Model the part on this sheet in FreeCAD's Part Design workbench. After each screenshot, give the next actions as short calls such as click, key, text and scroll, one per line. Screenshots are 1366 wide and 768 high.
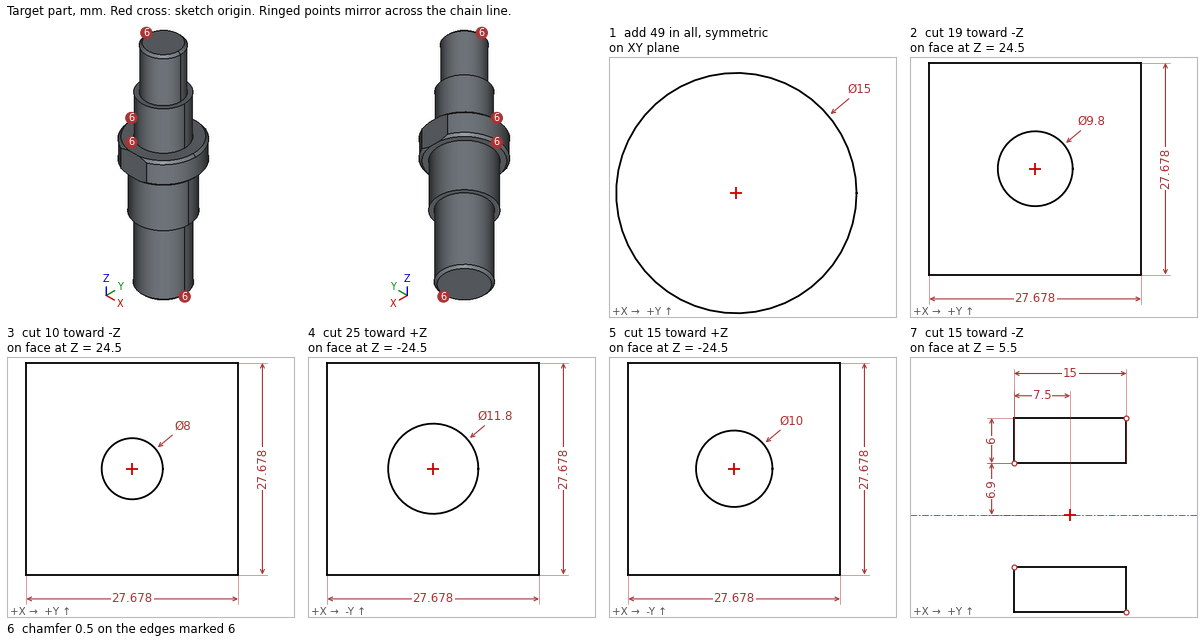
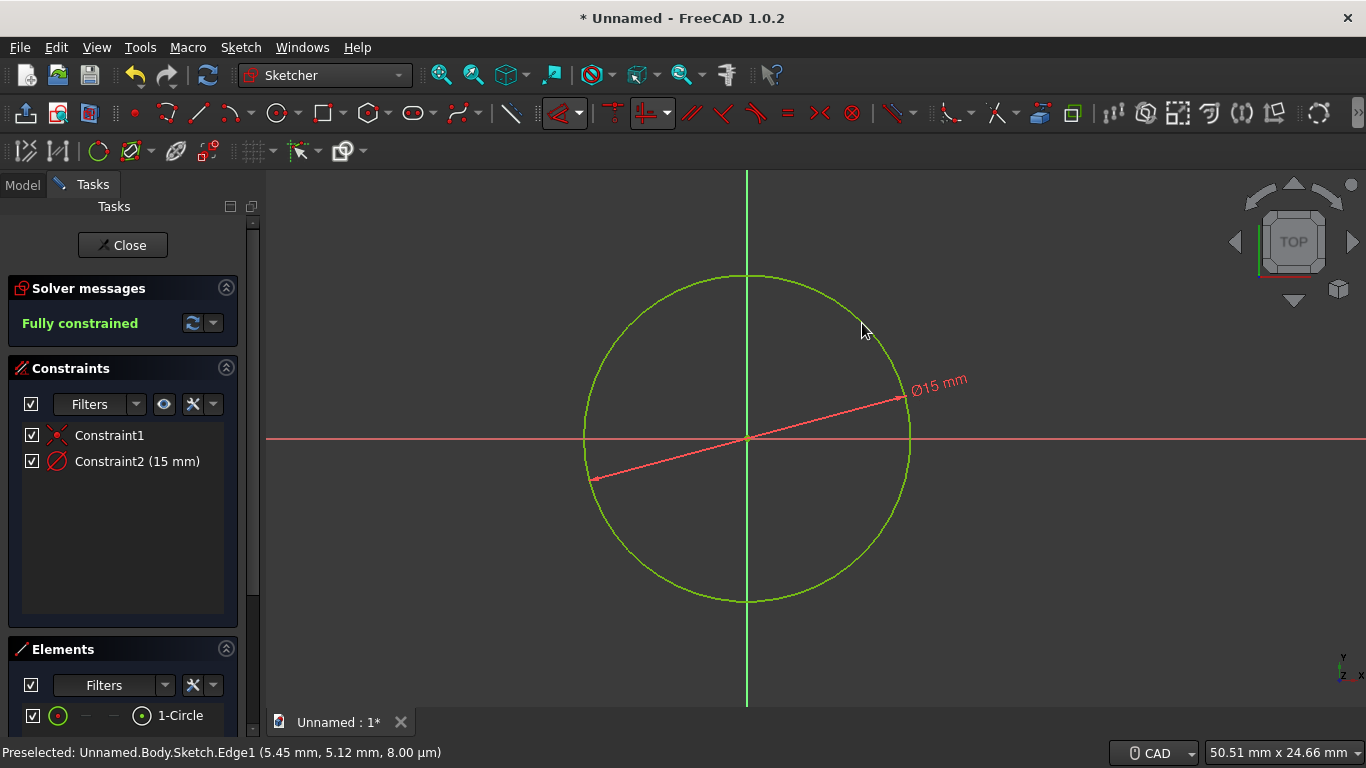
click(123, 245)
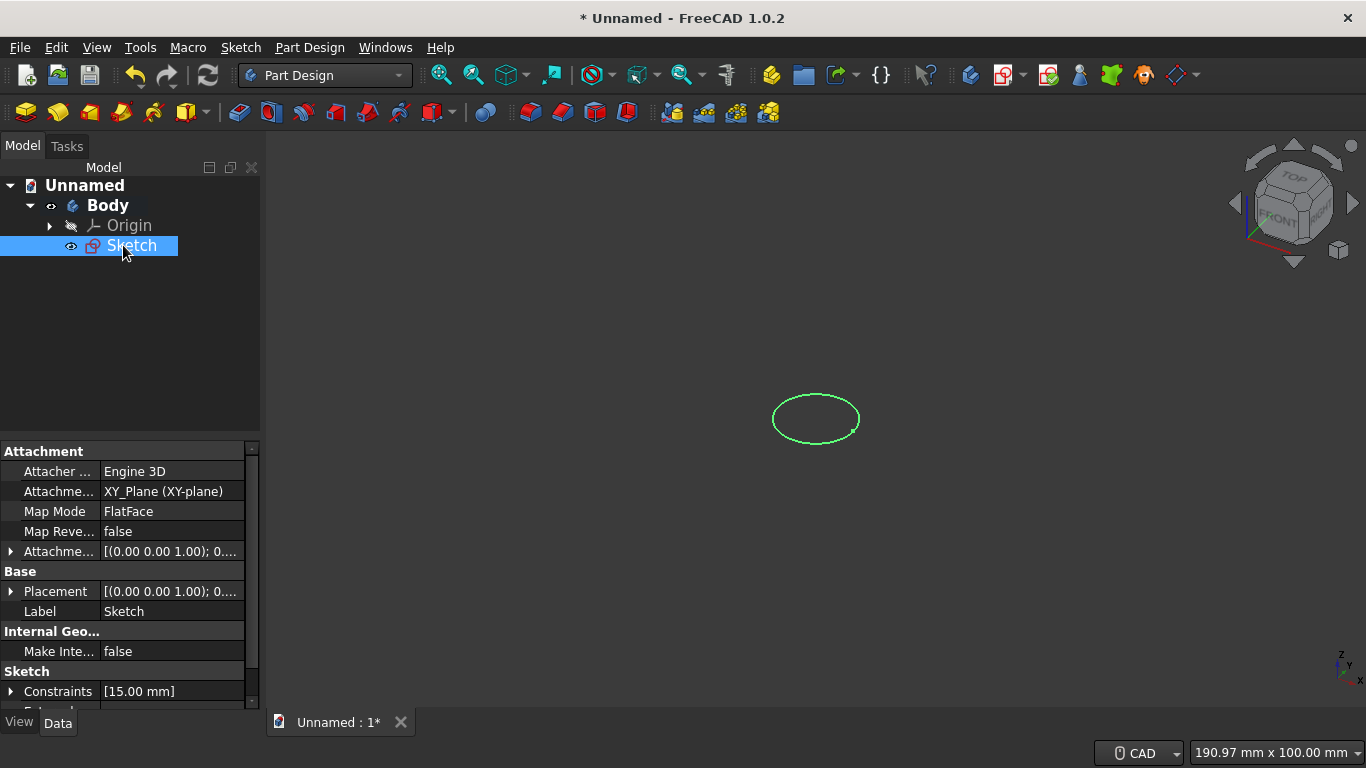
click(26, 112)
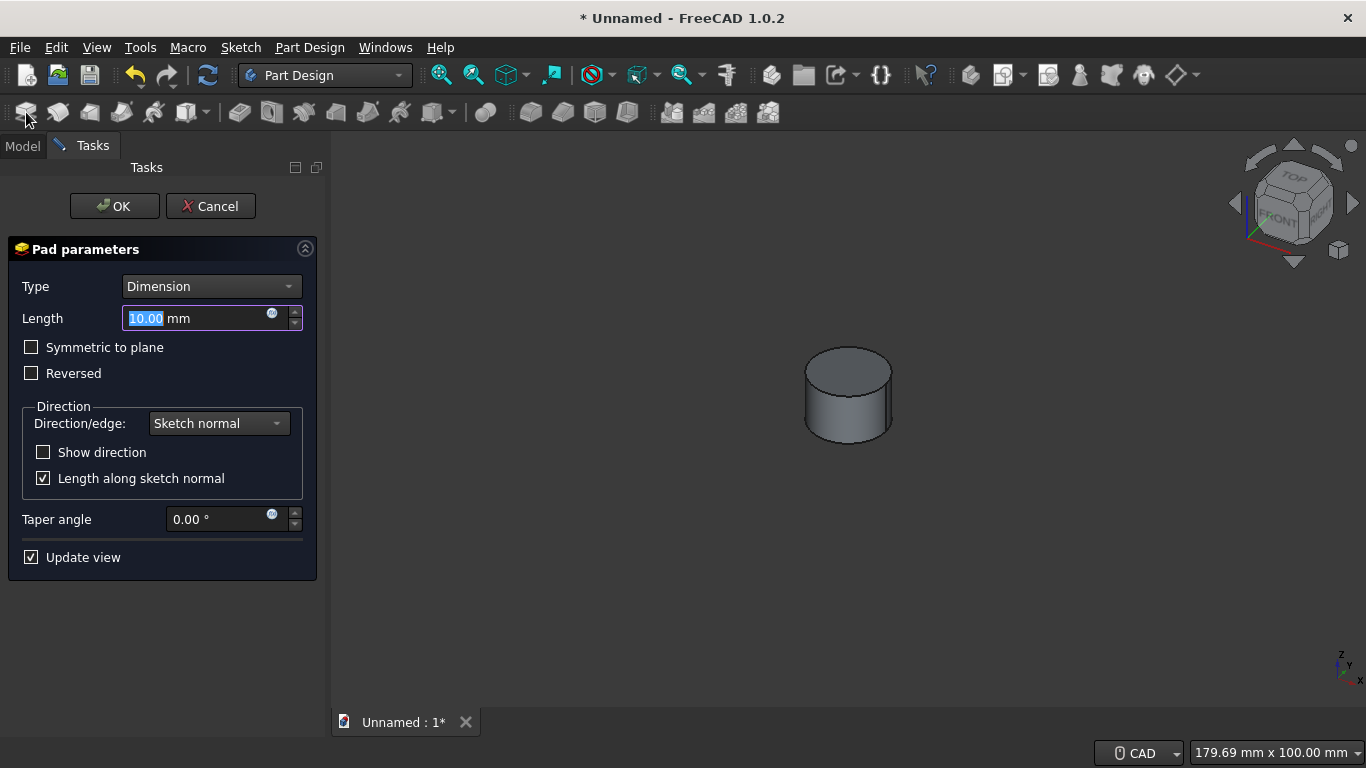
text(49)
key(Tab)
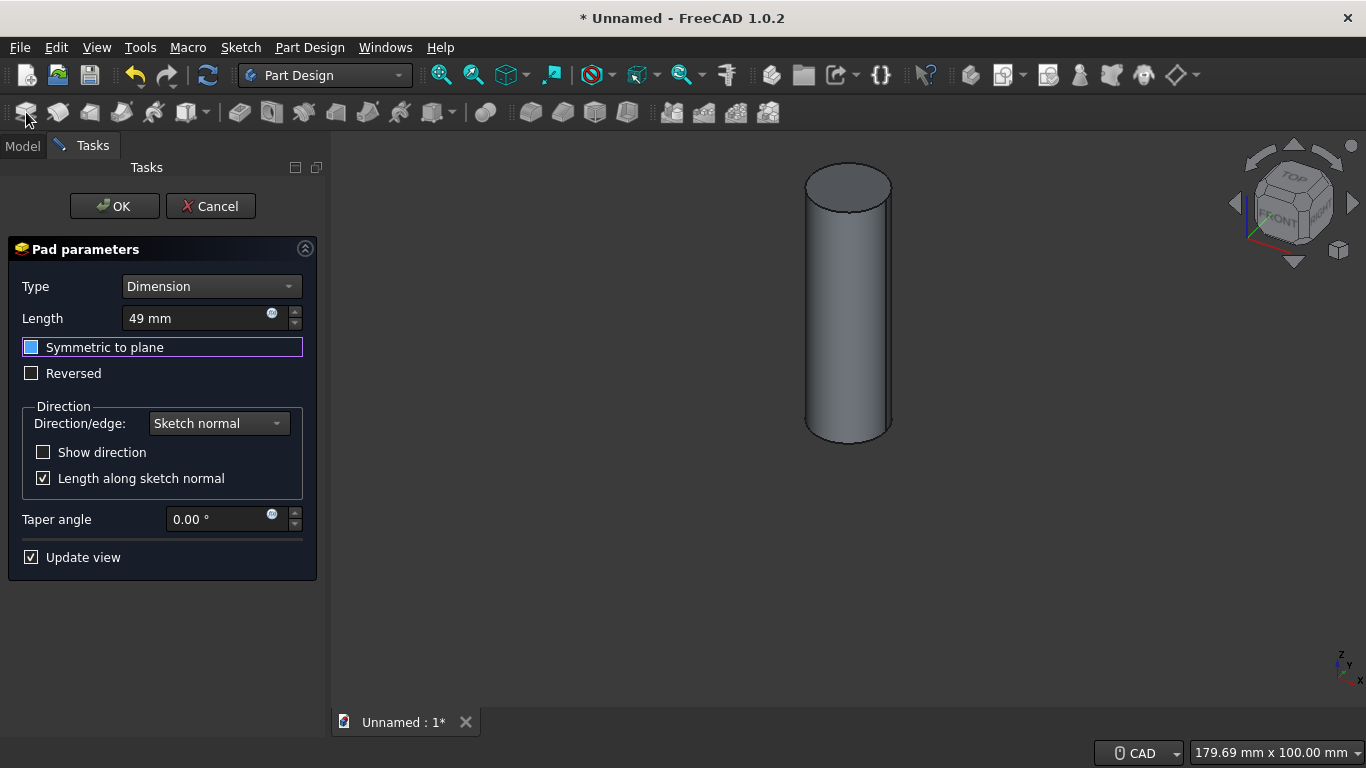
click(30, 347)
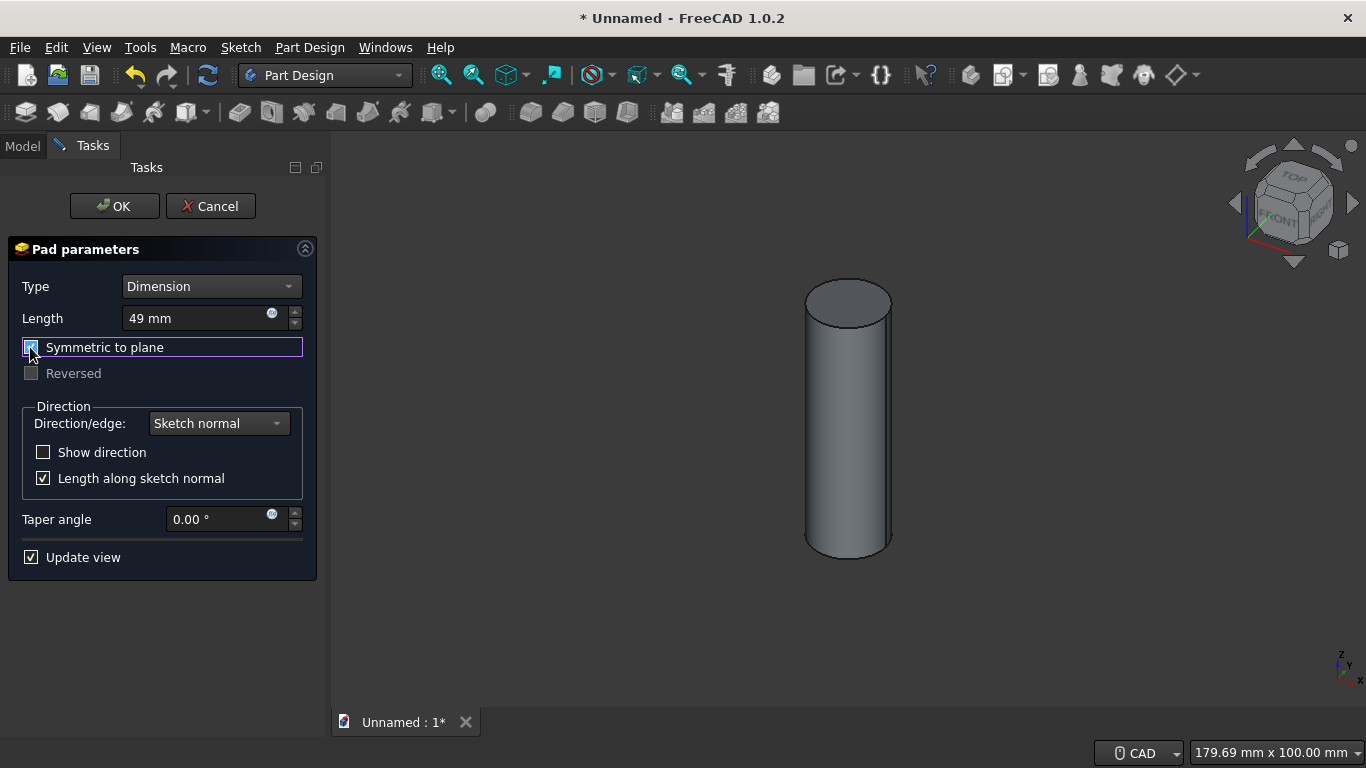
click(115, 206)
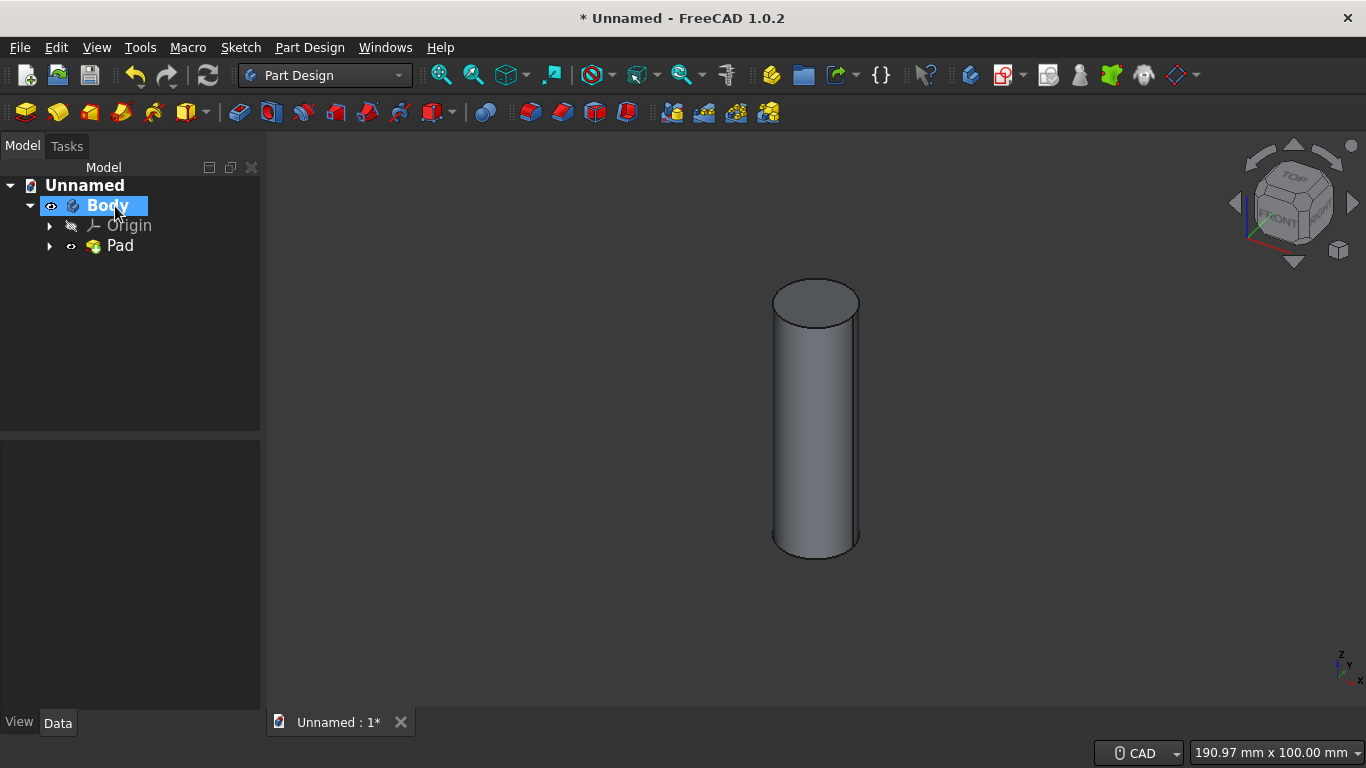
click(816, 302)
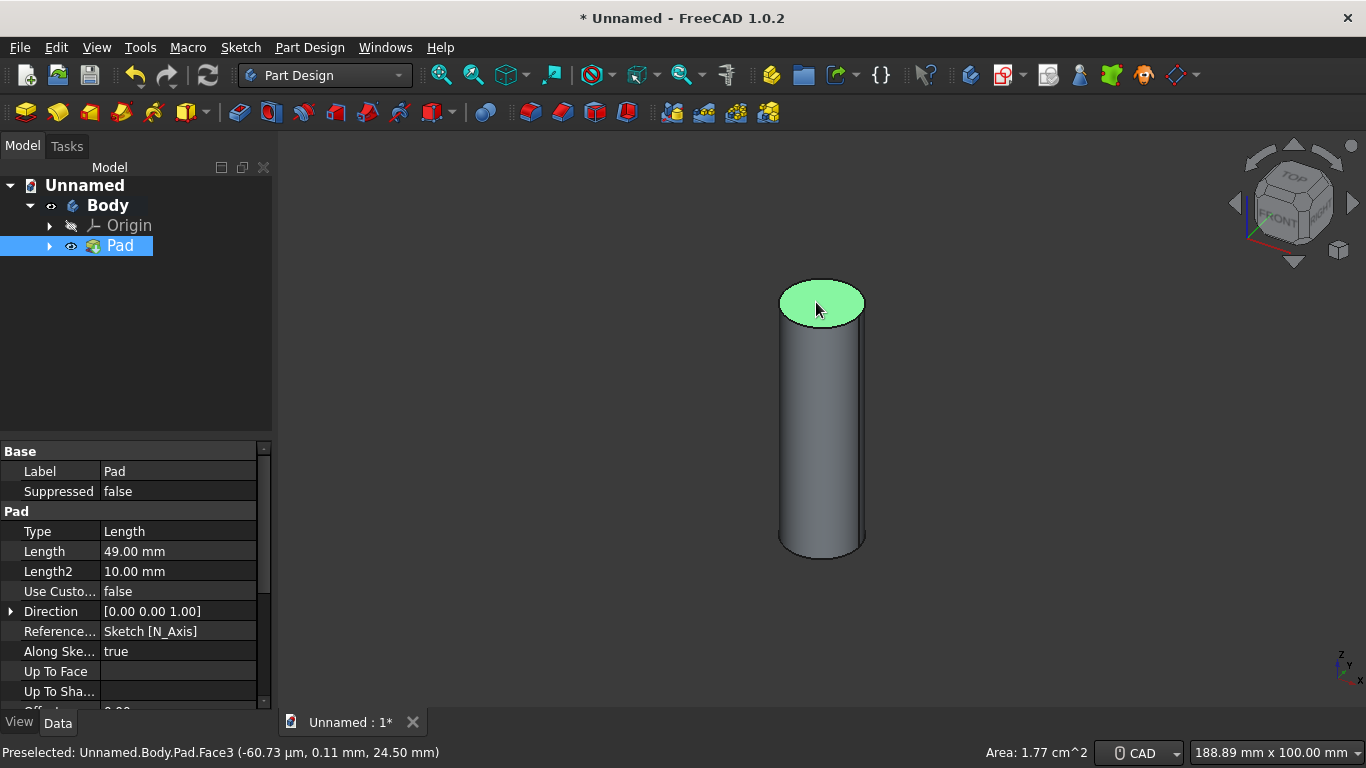
click(1004, 76)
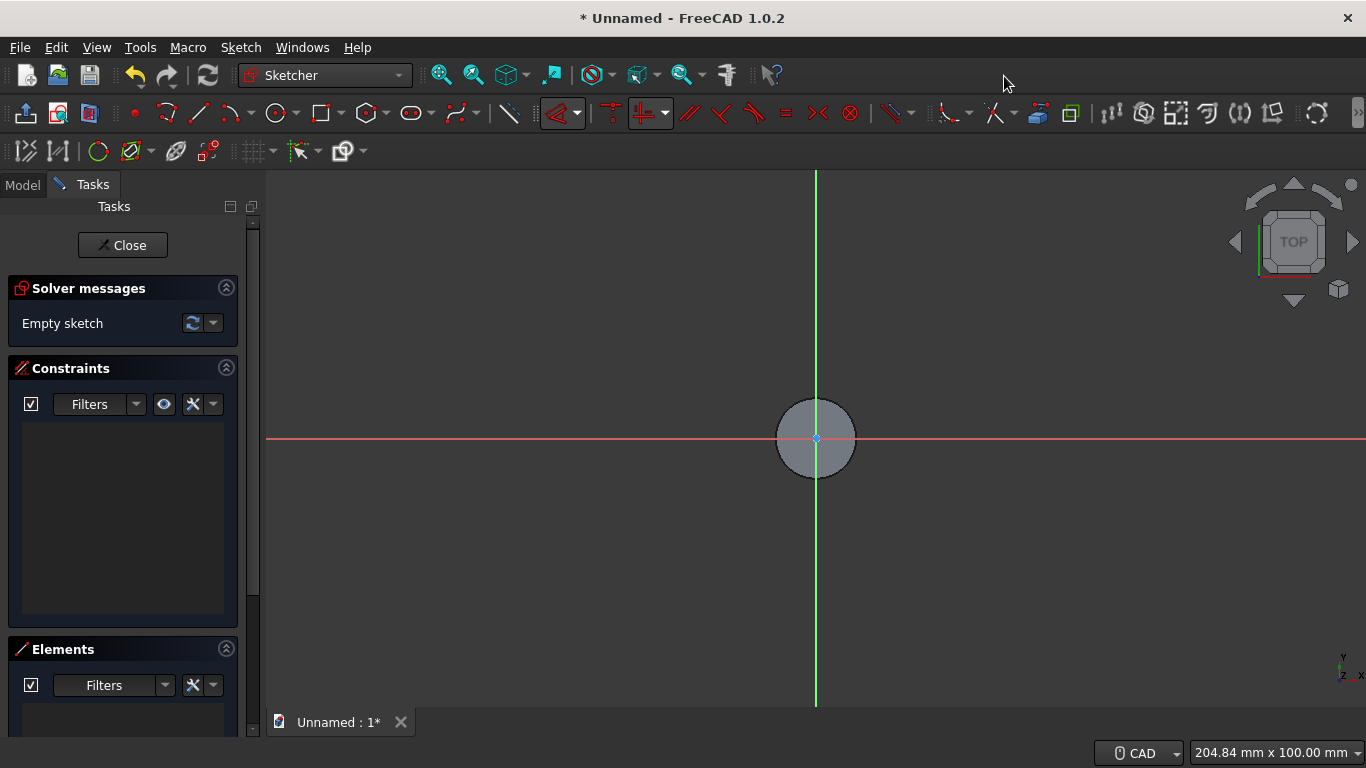
scroll(872, 438, up, 4)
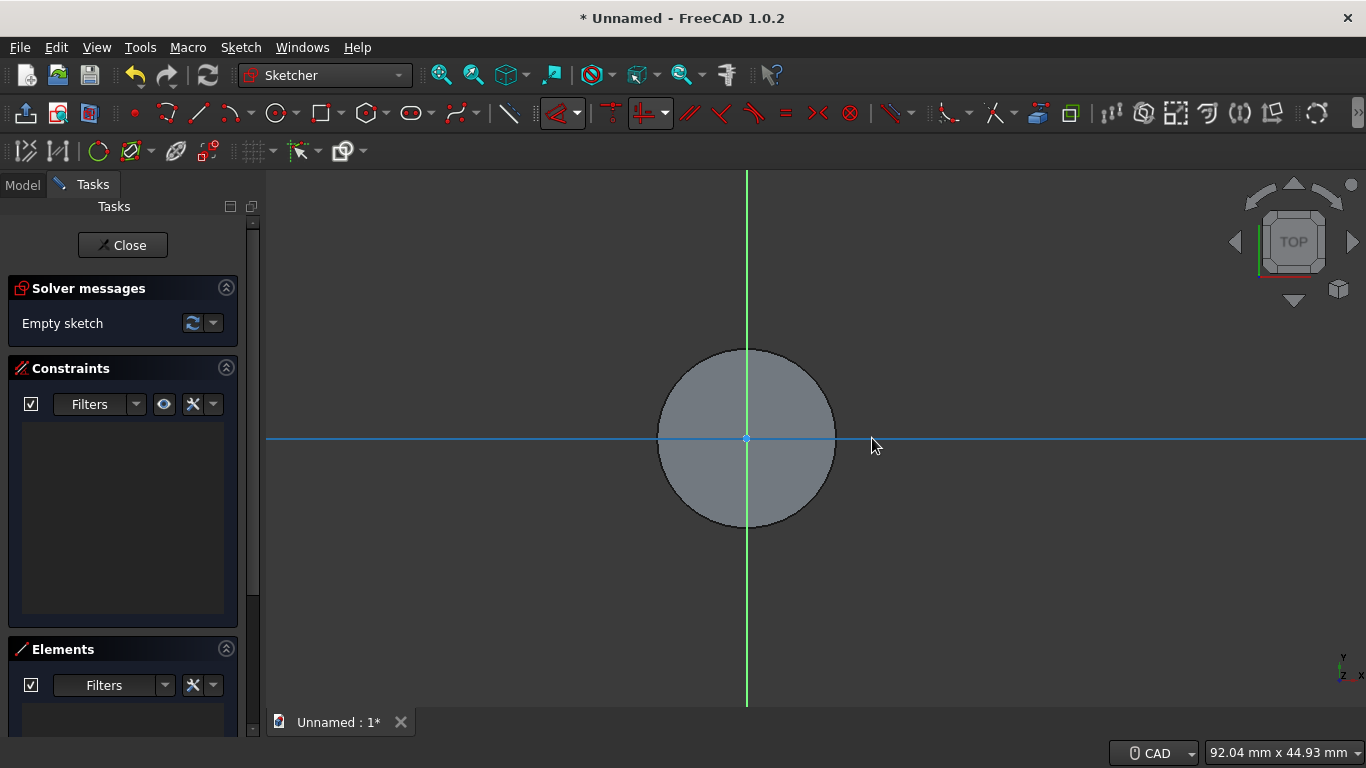
click(344, 114)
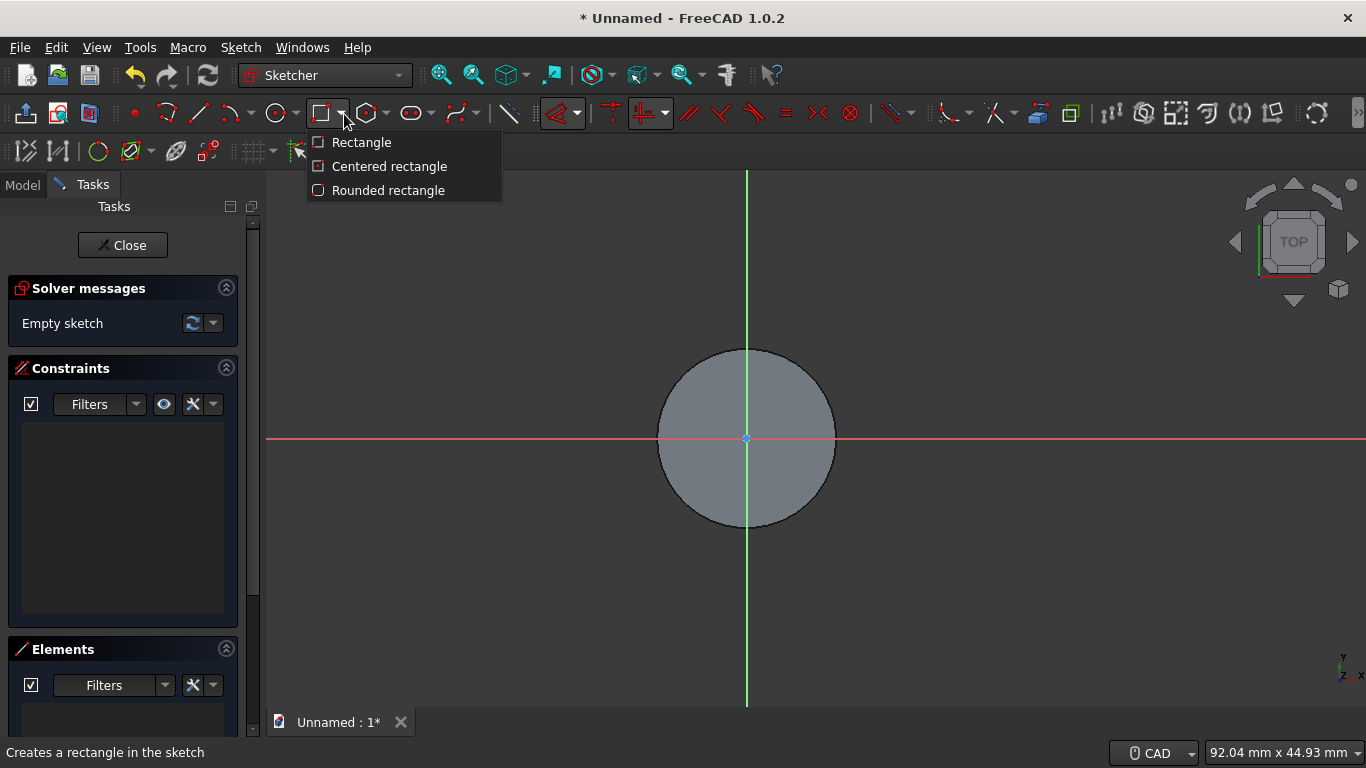
click(404, 166)